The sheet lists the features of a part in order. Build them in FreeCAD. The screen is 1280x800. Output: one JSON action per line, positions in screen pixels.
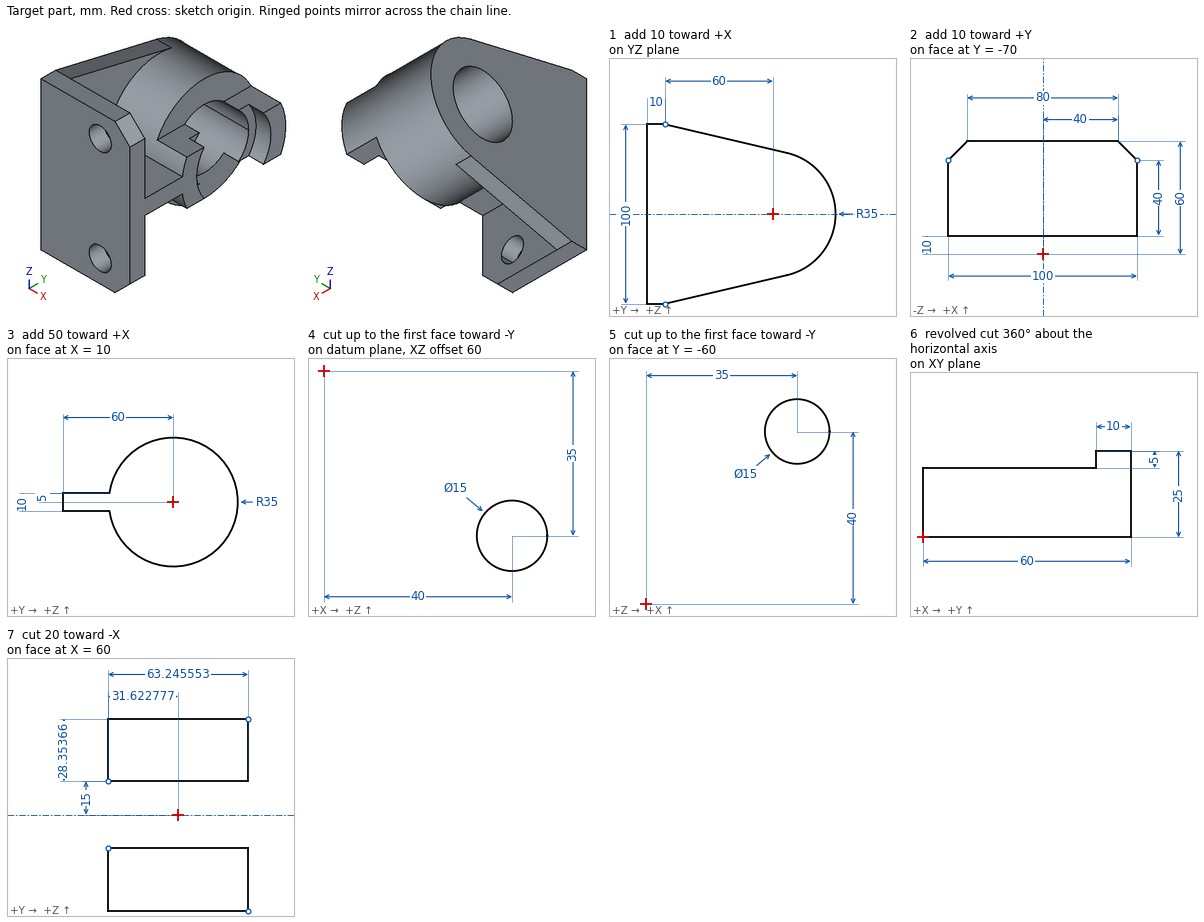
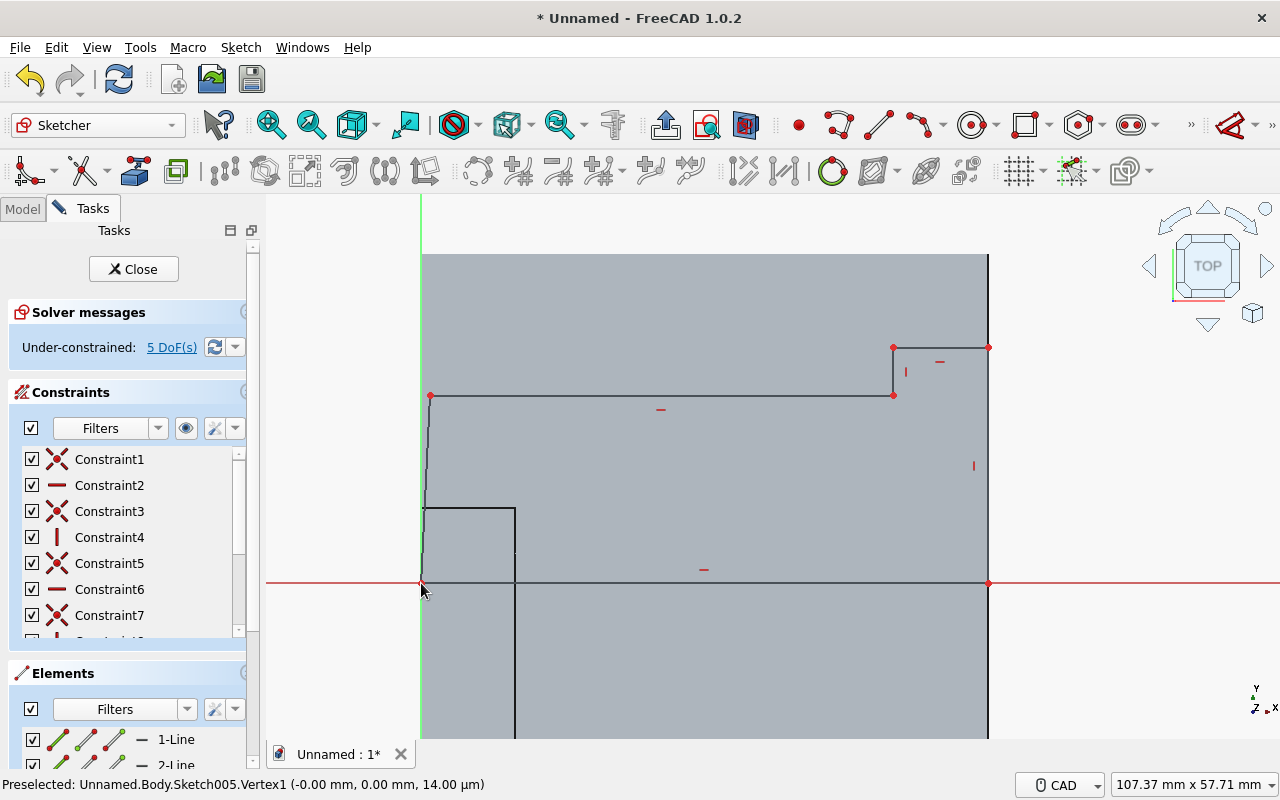
{"action": "left_click", "coordinate": [424, 527]}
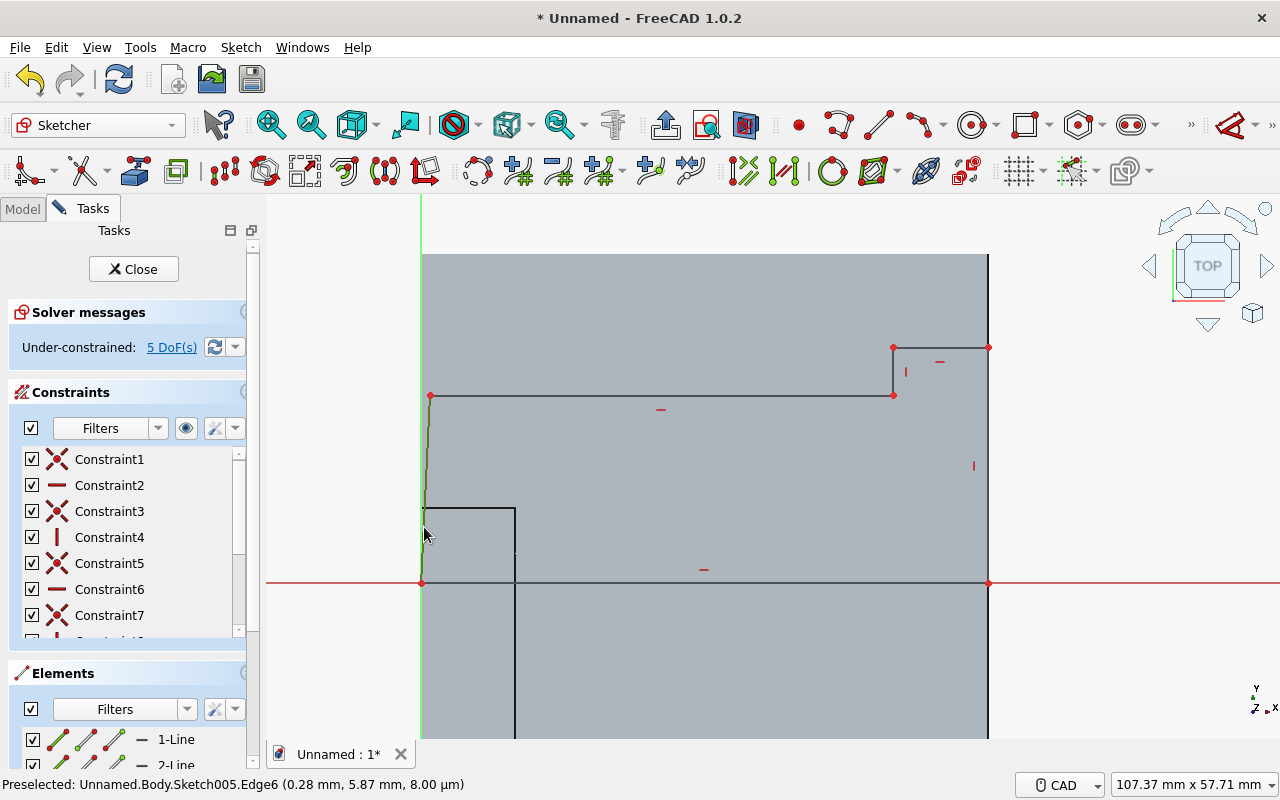
{"action": "key", "text": "v"}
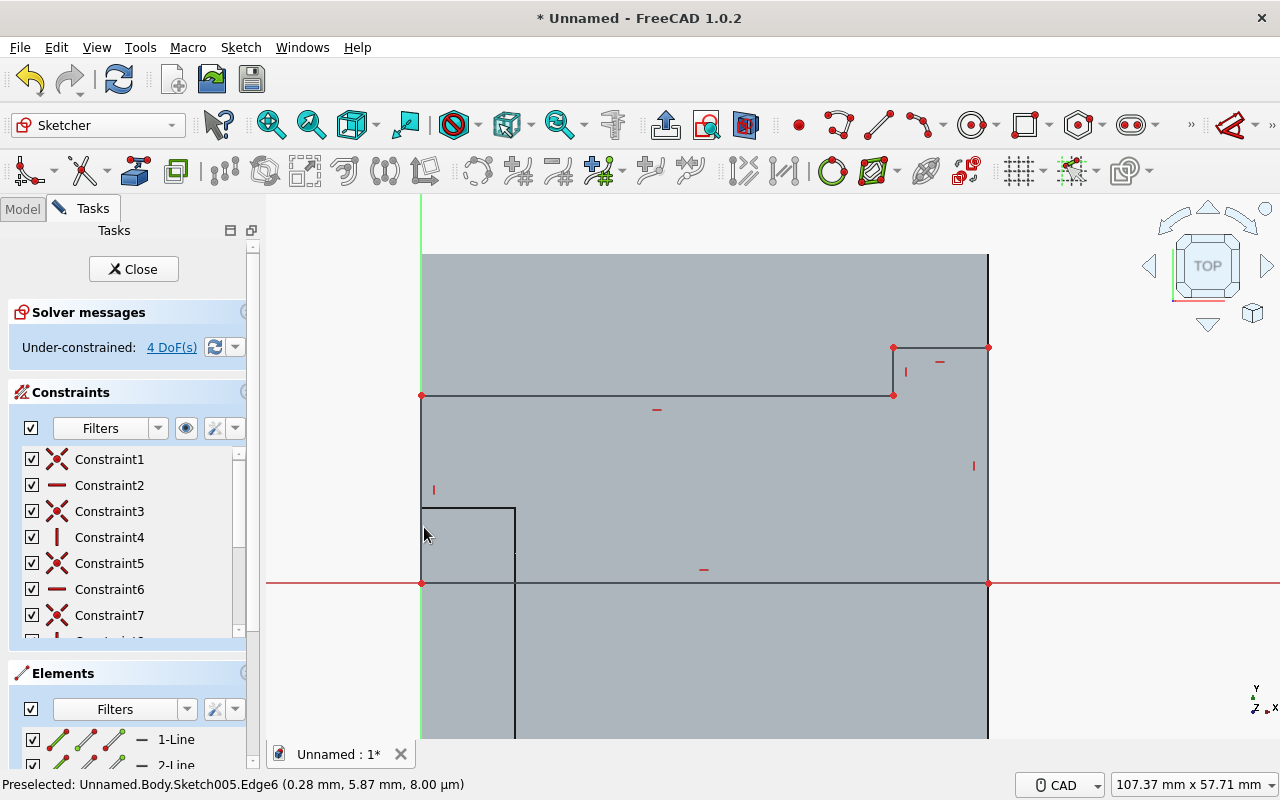
{"action": "left_click", "coordinate": [1230, 126]}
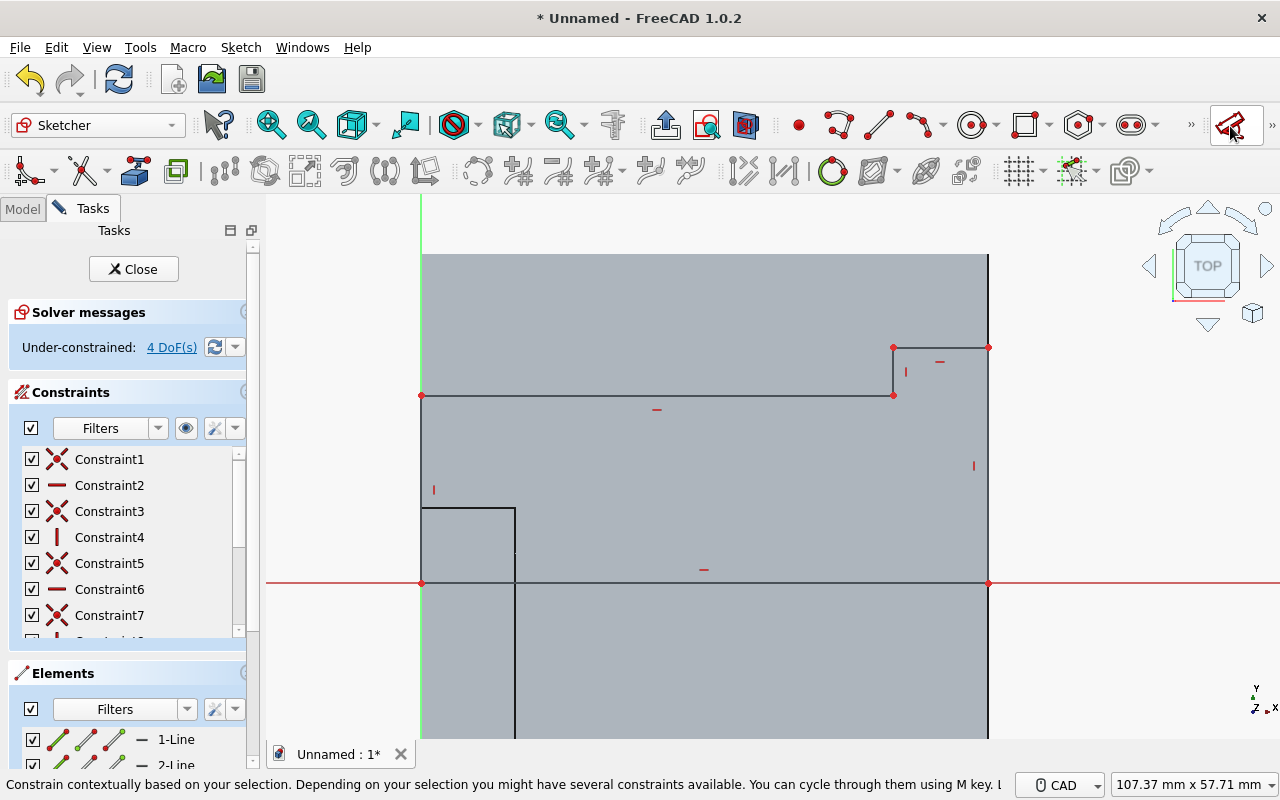
{"action": "left_click", "coordinate": [893, 362]}
{"action": "left_click", "coordinate": [927, 372]}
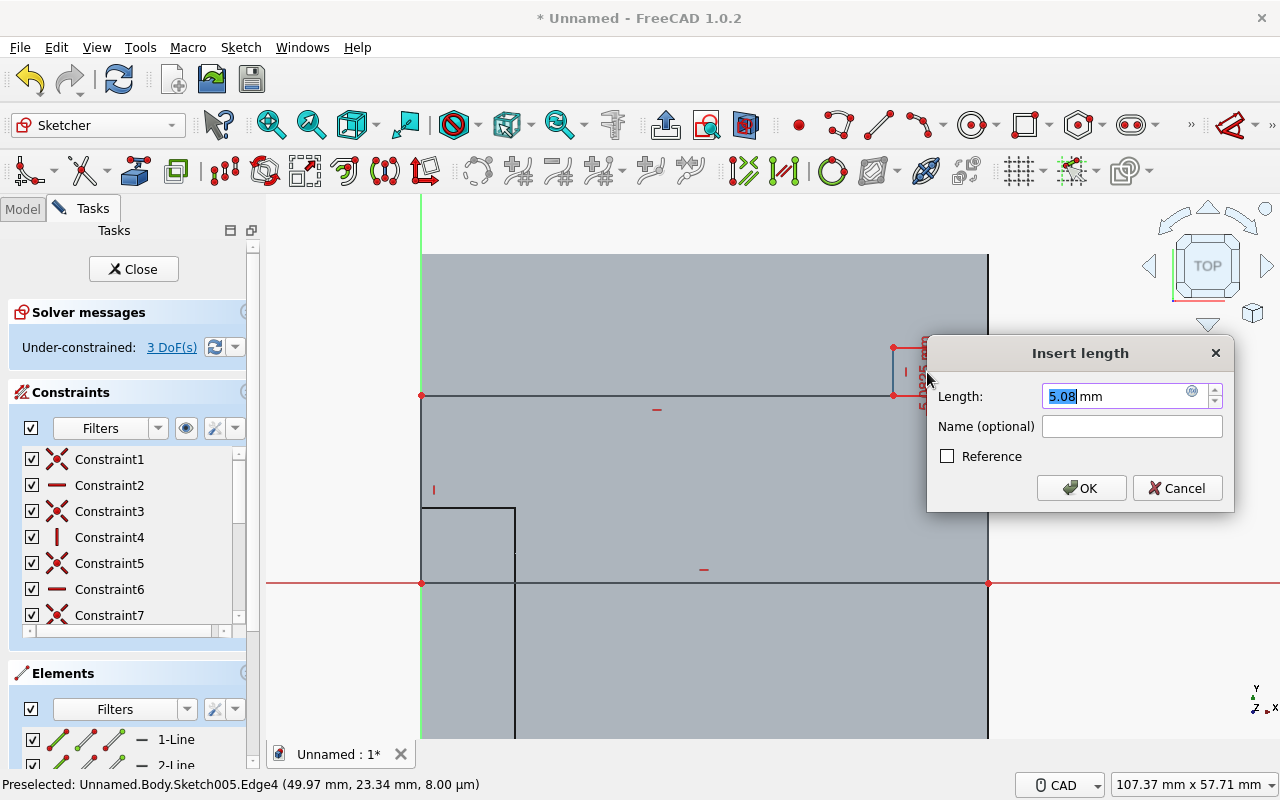
{"action": "type", "text": "5"}
{"action": "key", "text": "Return"}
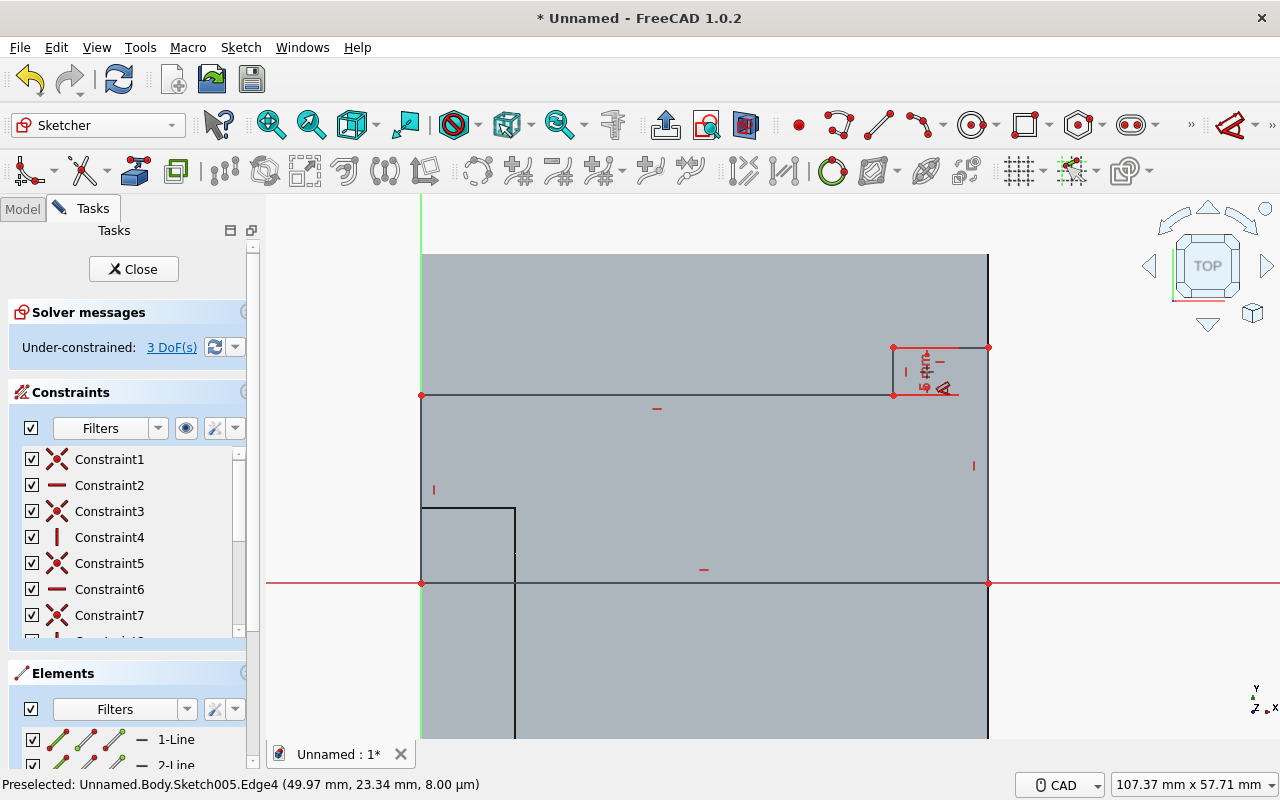
{"action": "left_click", "coordinate": [591, 583]}
{"action": "left_click", "coordinate": [705, 617]}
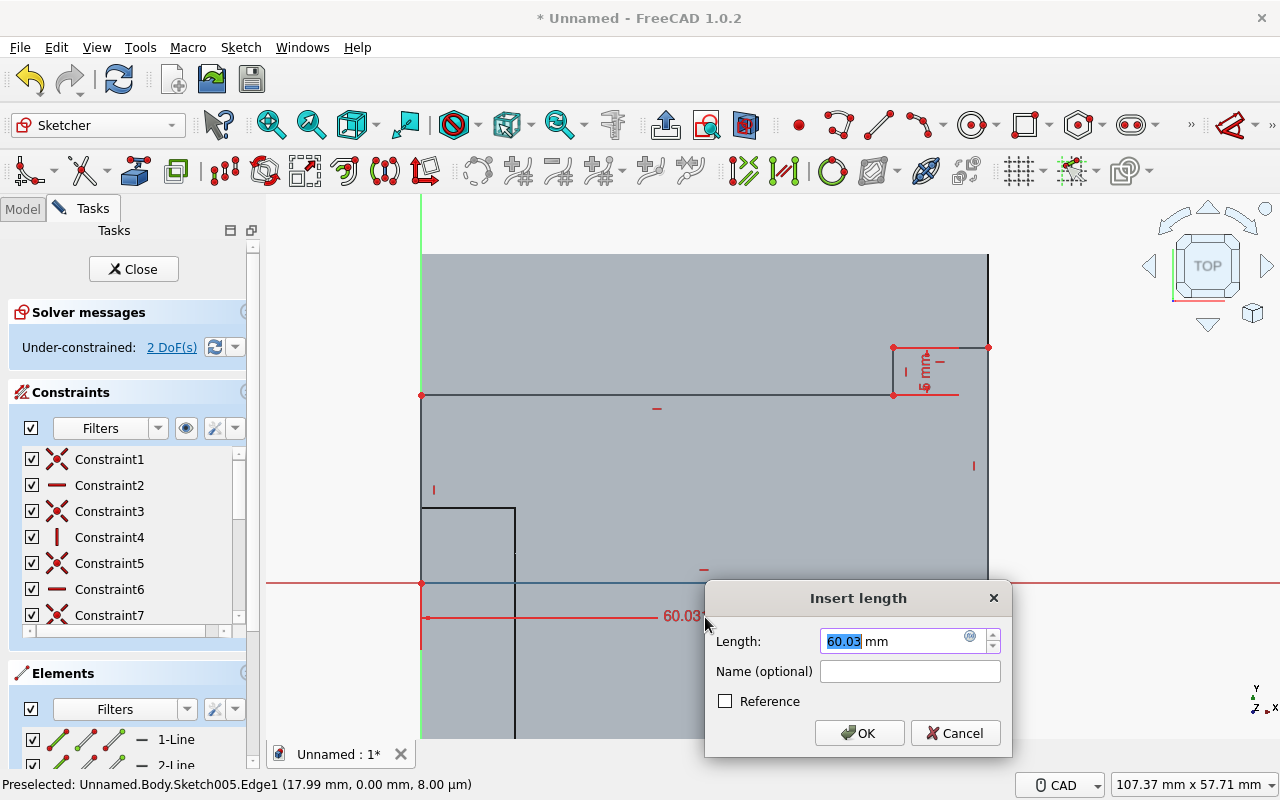
{"action": "type", "text": "60"}
{"action": "key", "text": "Return"}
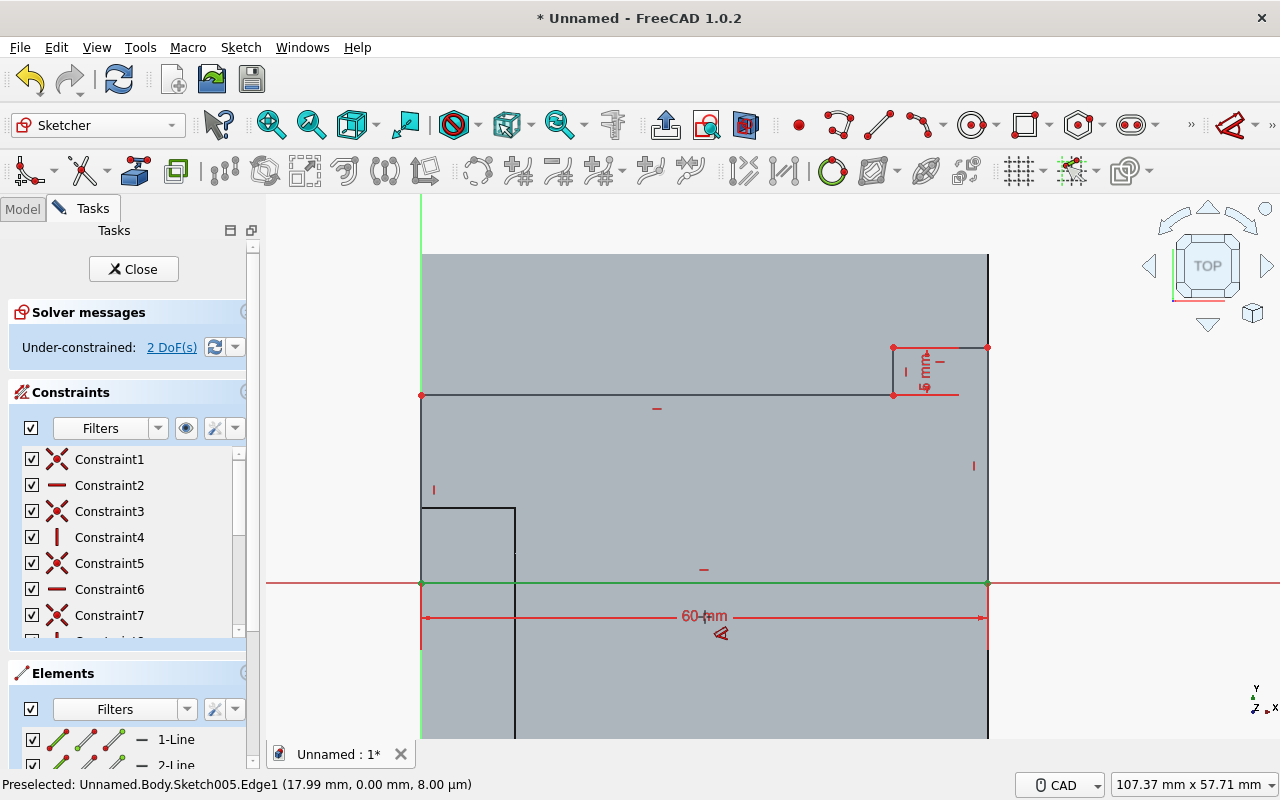
{"action": "left_click", "coordinate": [988, 513]}
{"action": "left_click", "coordinate": [1022, 466]}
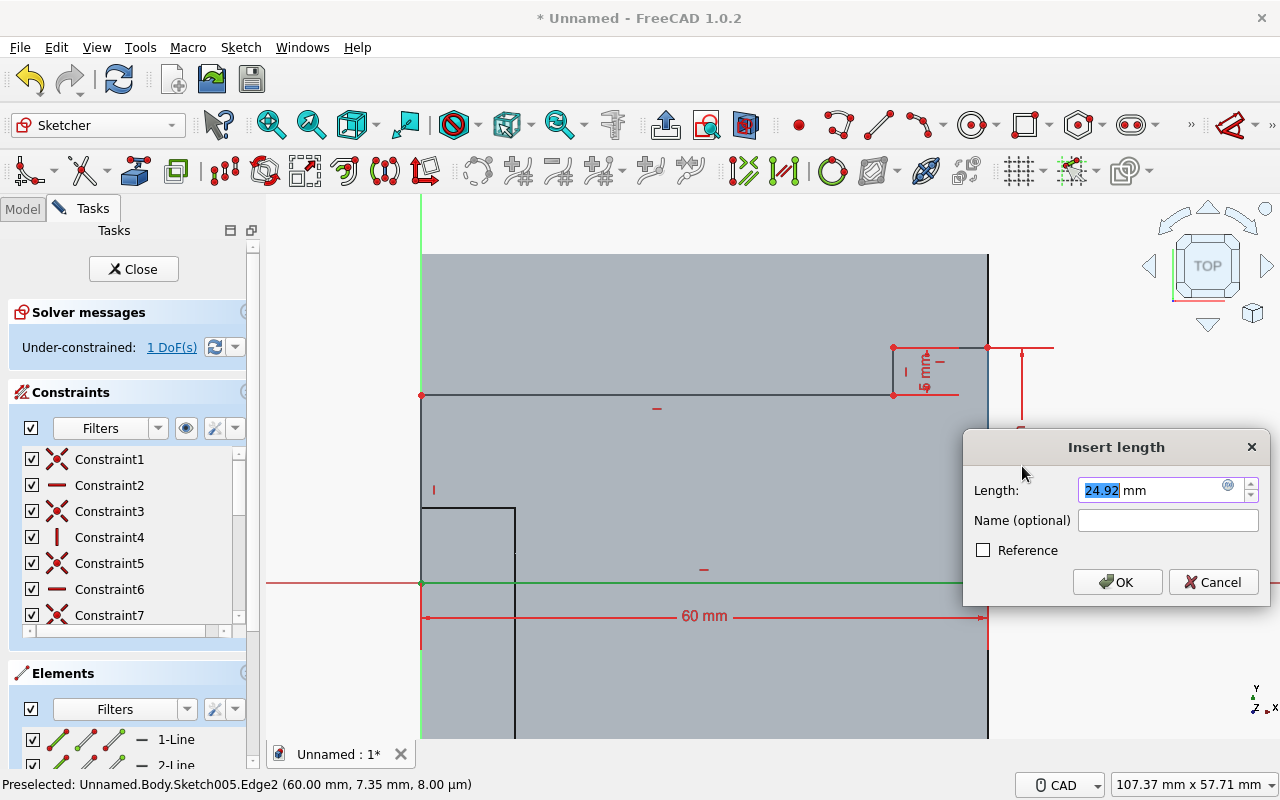
{"action": "type", "text": "25"}
{"action": "key", "text": "Return"}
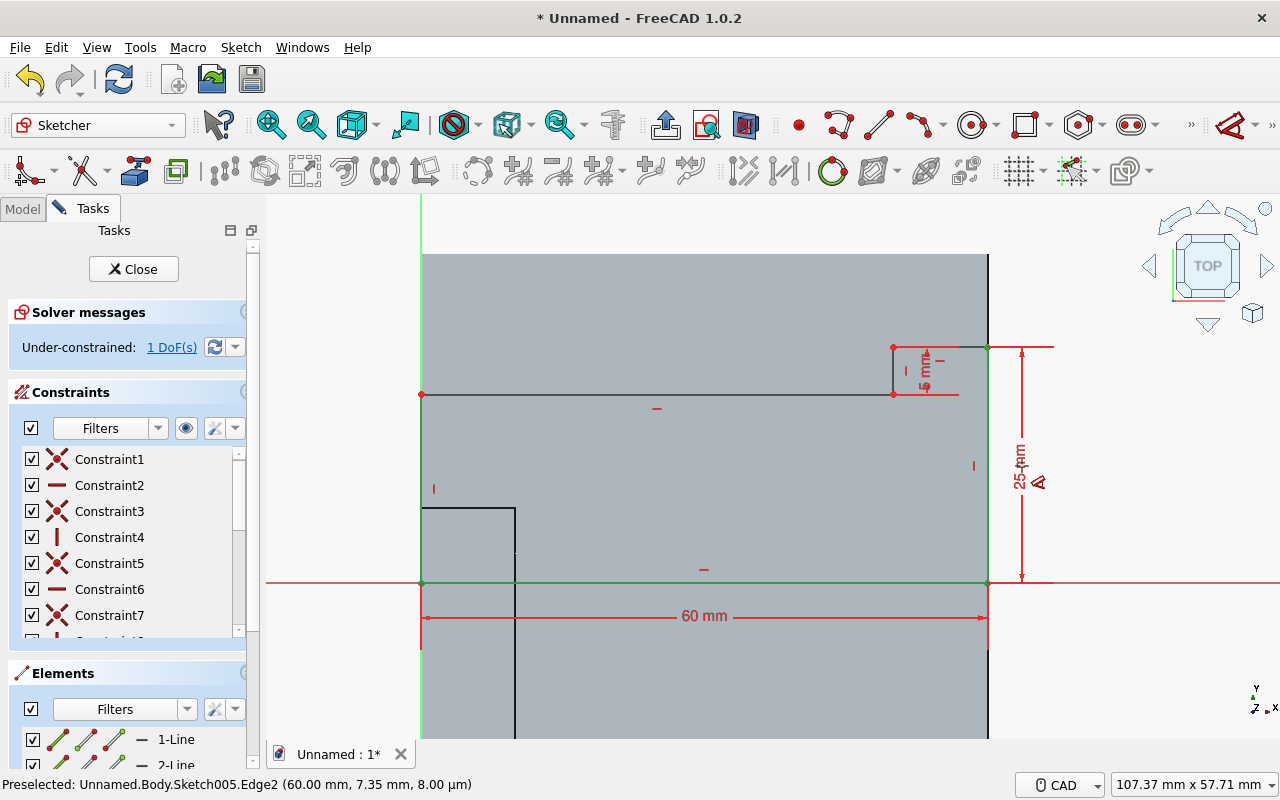
{"action": "left_click", "coordinate": [959, 347]}
{"action": "left_click", "coordinate": [940, 313]}